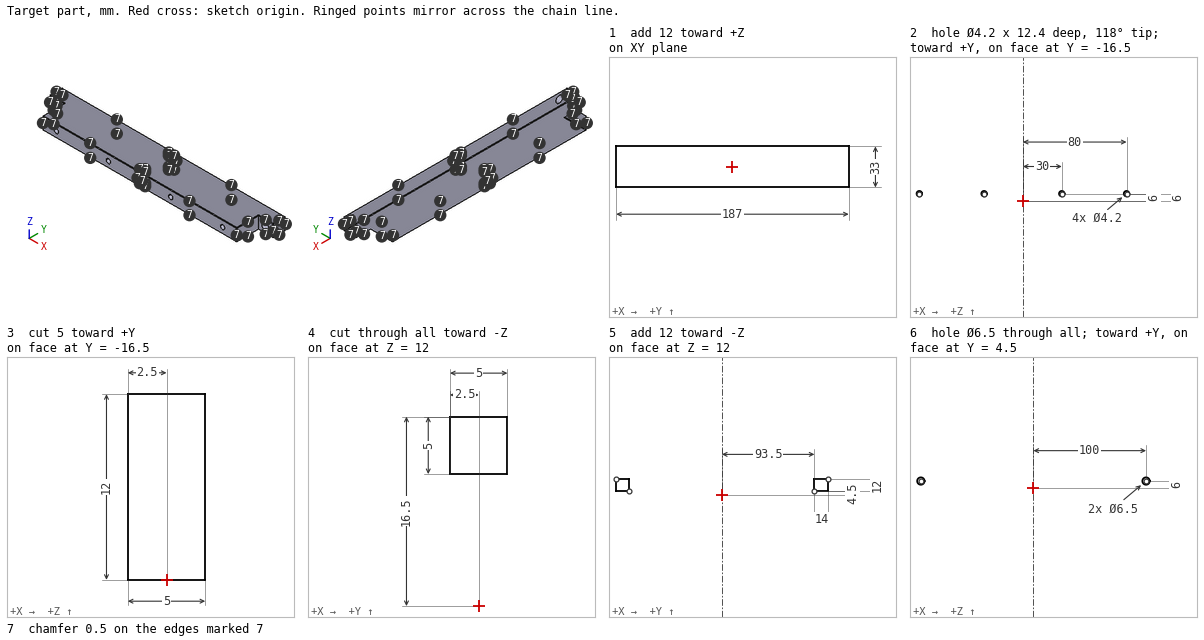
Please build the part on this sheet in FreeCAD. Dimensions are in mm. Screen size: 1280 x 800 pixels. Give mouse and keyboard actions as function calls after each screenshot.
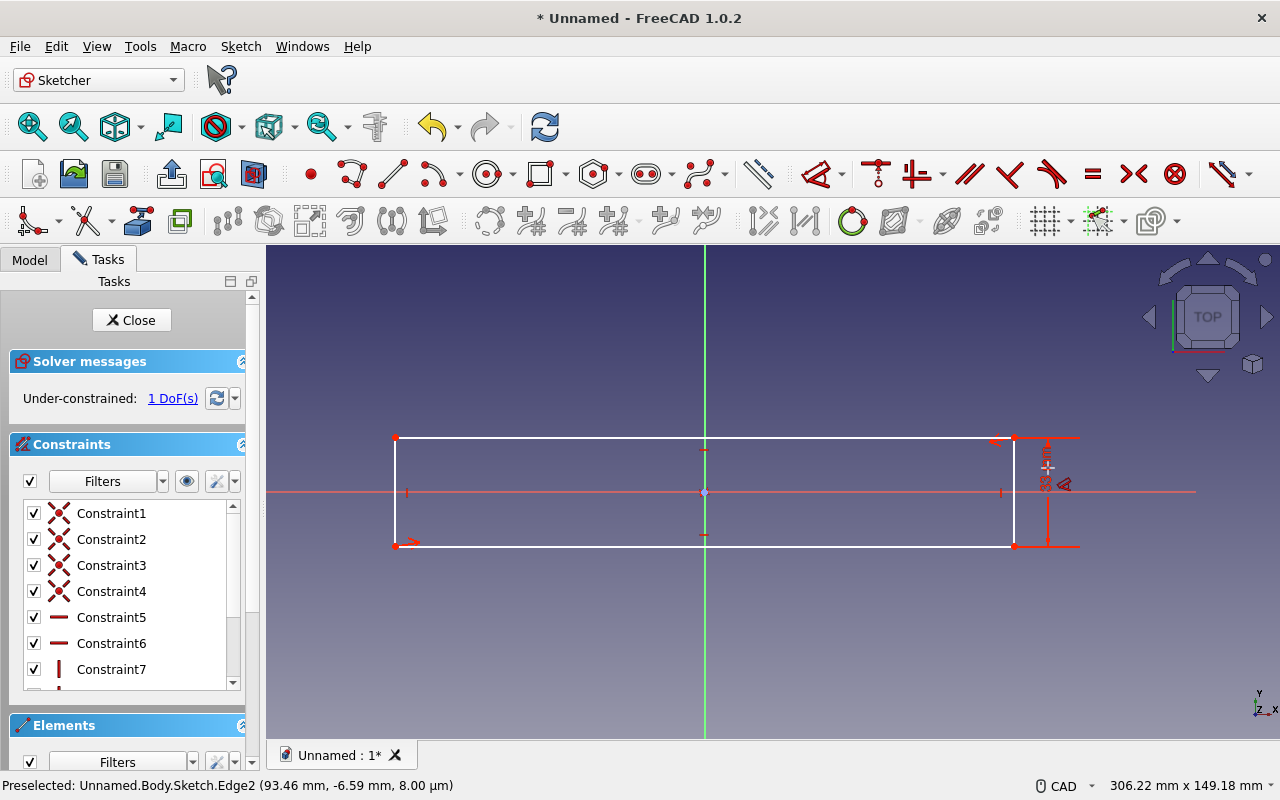
click(581, 547)
click(562, 581)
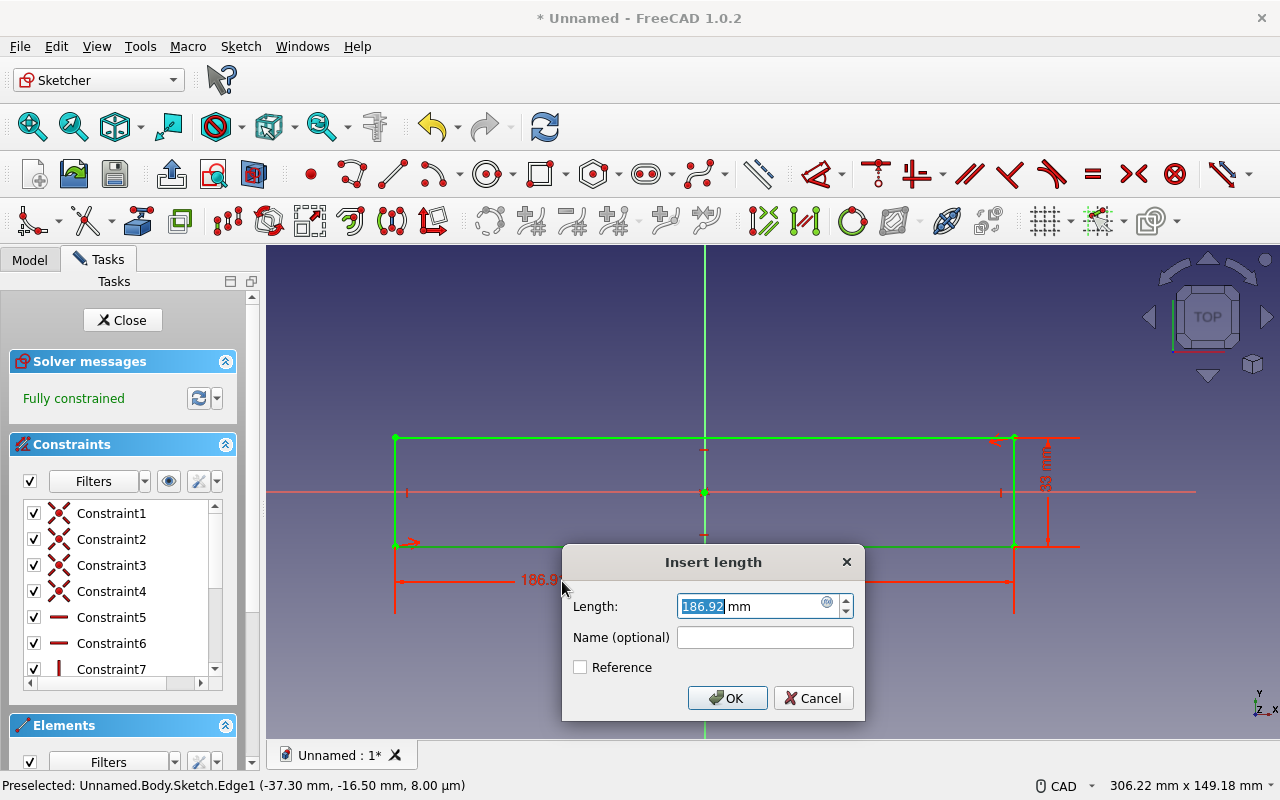
text(187)
key(Return)
key(Escape)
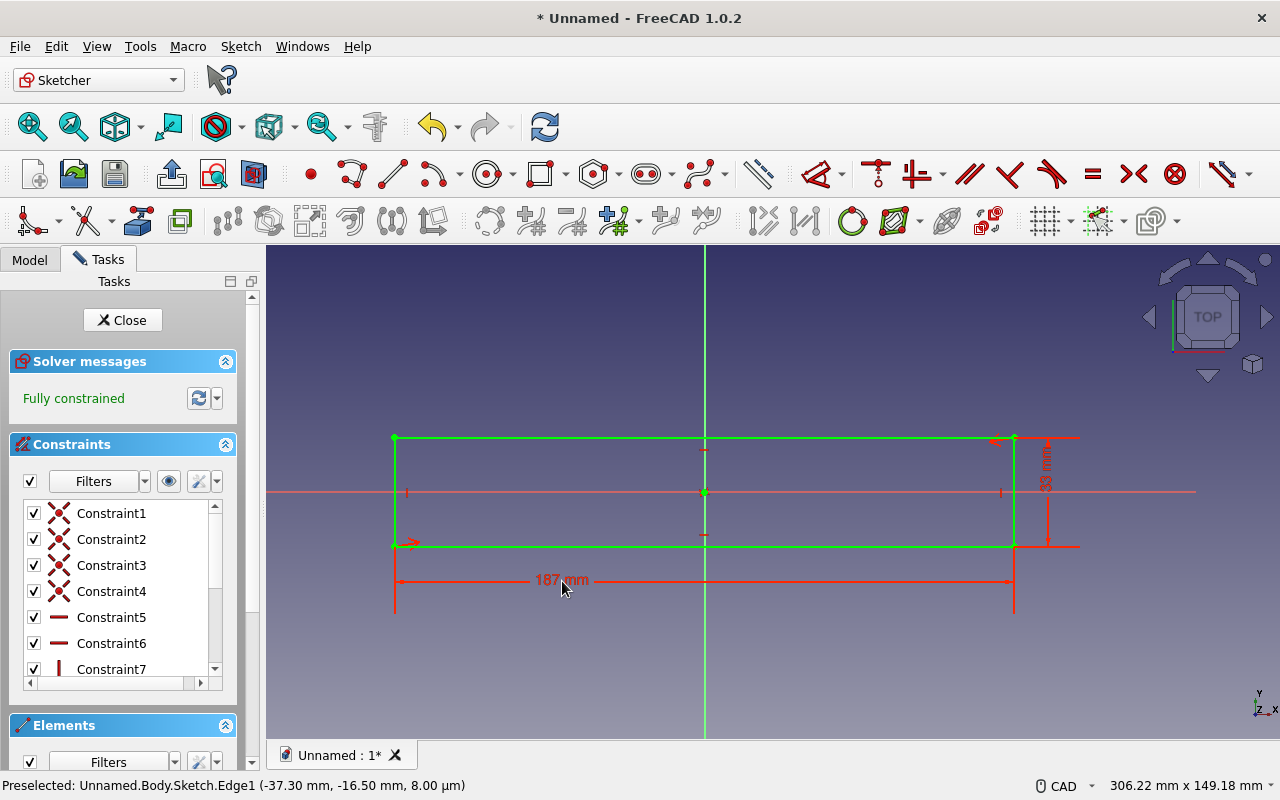
click(123, 320)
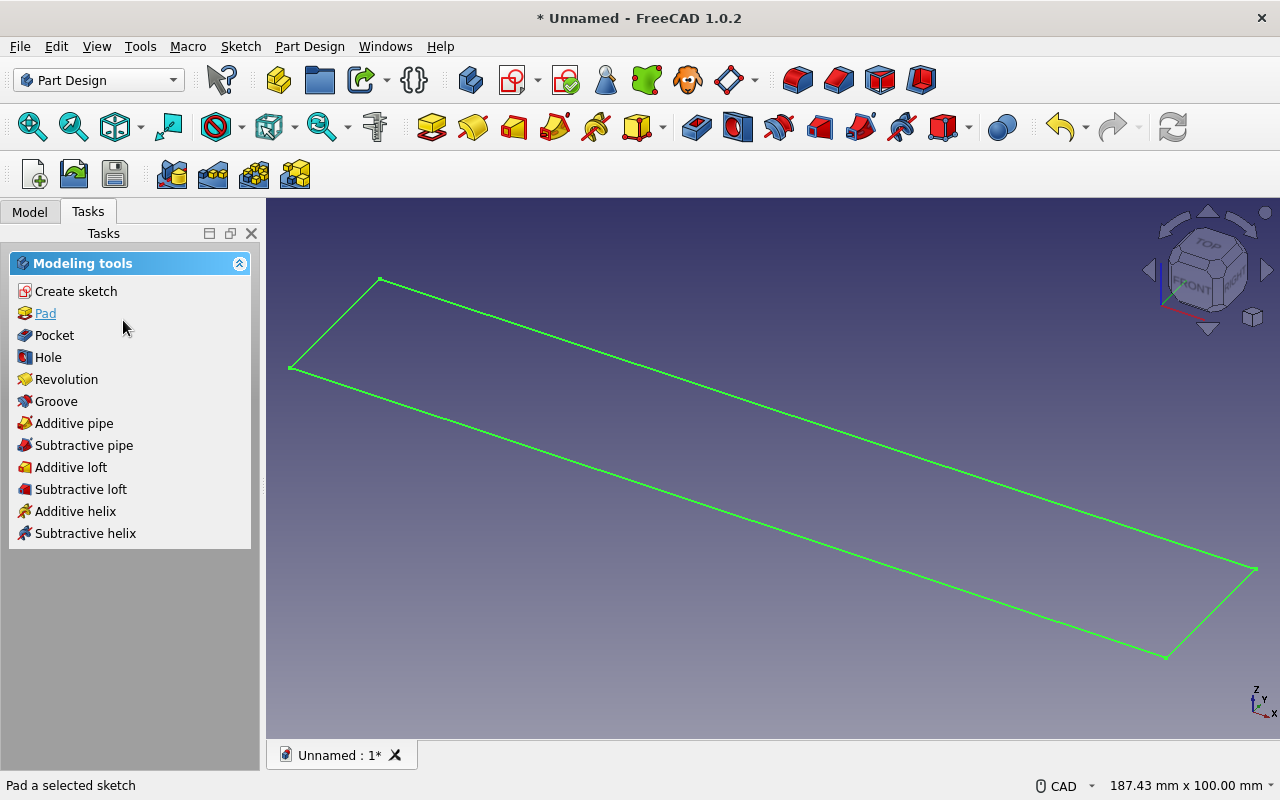
click(432, 128)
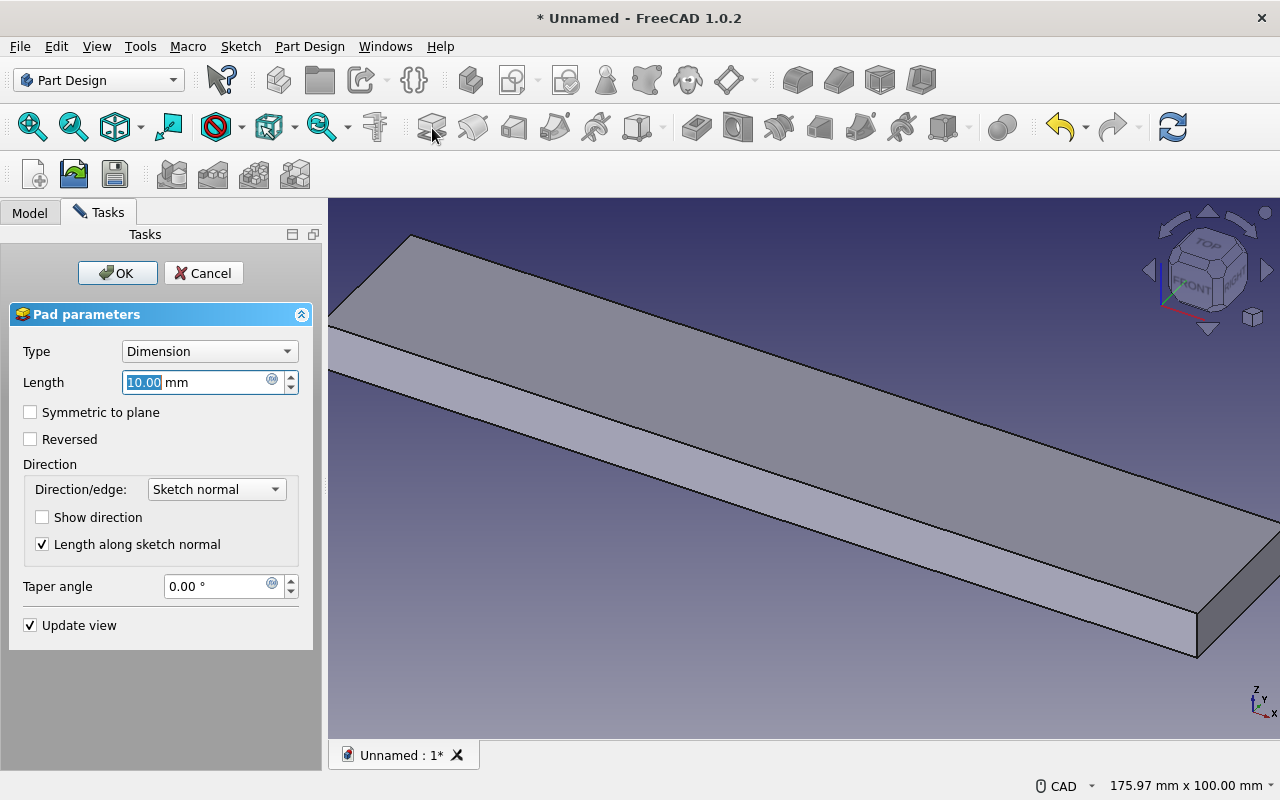
text(12)
key(Tab)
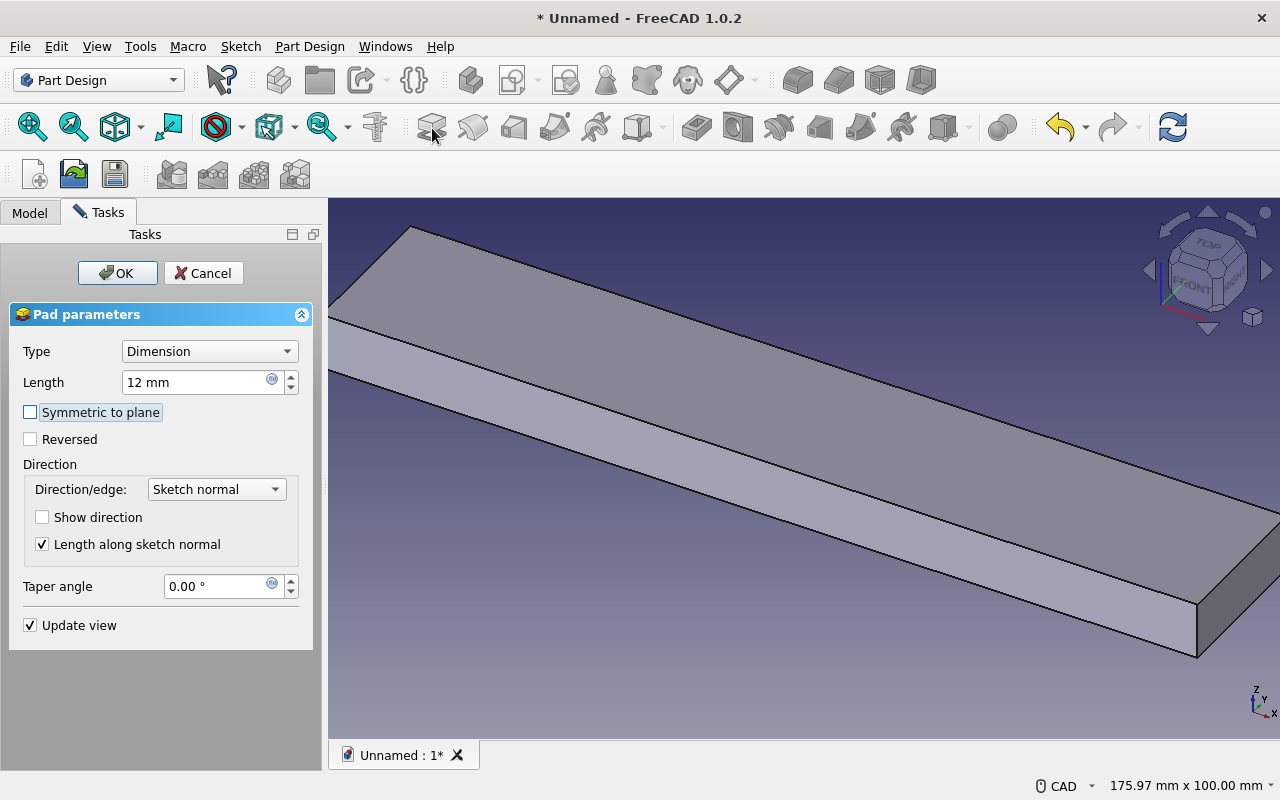
click(118, 273)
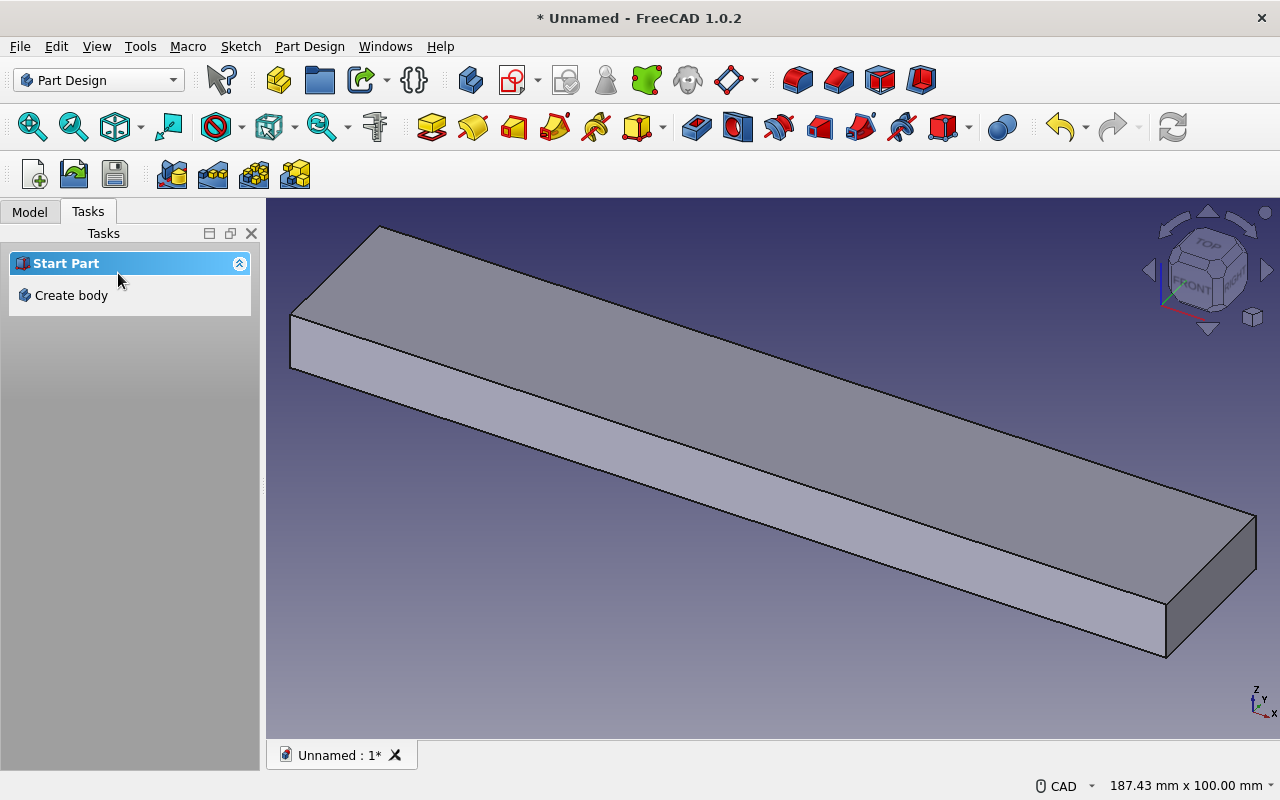
click(1104, 610)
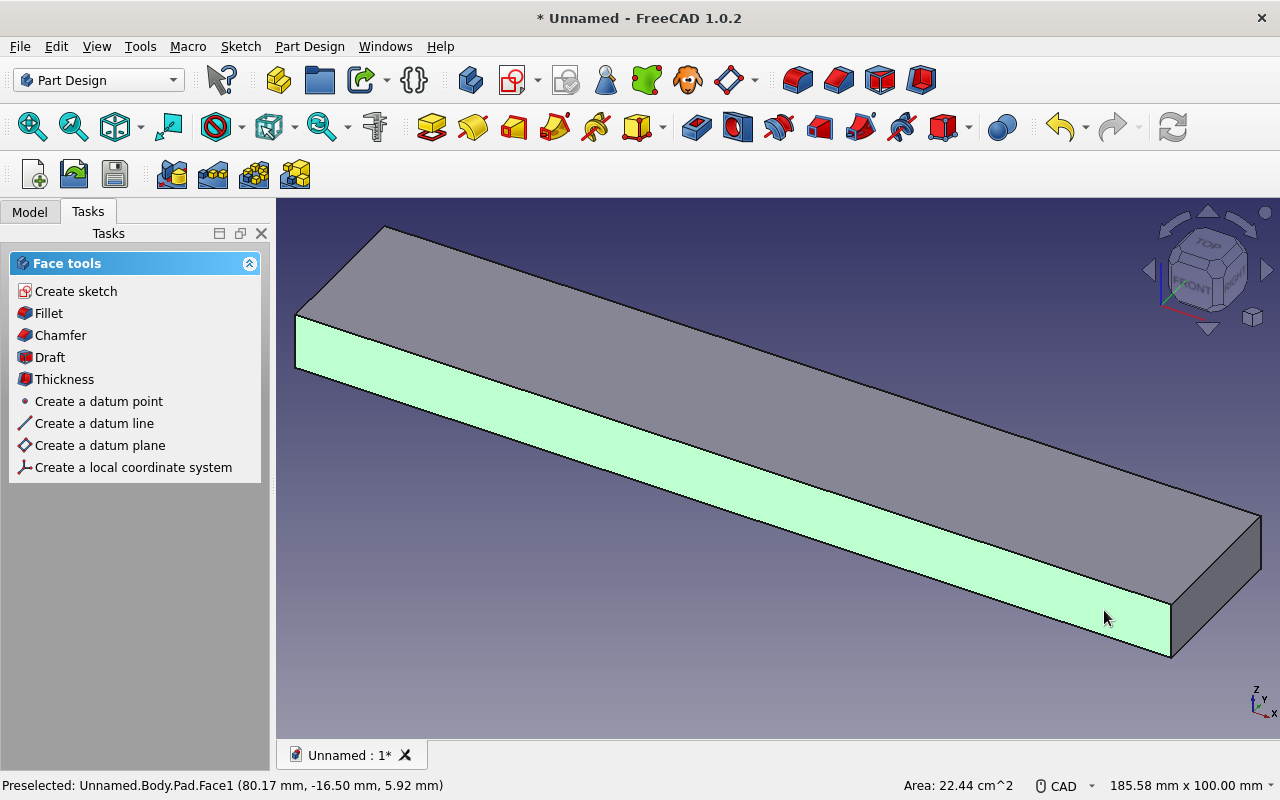
click(512, 80)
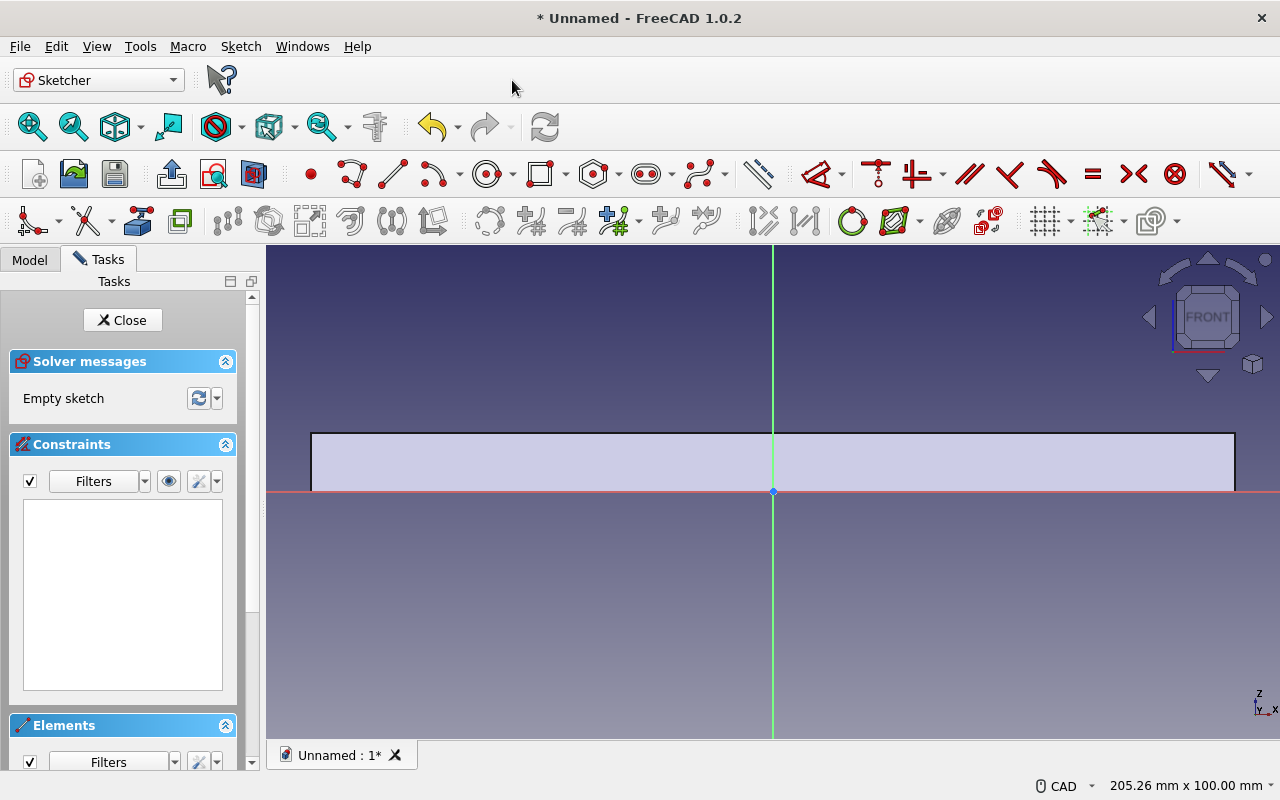
scroll(565, 533, down, 2)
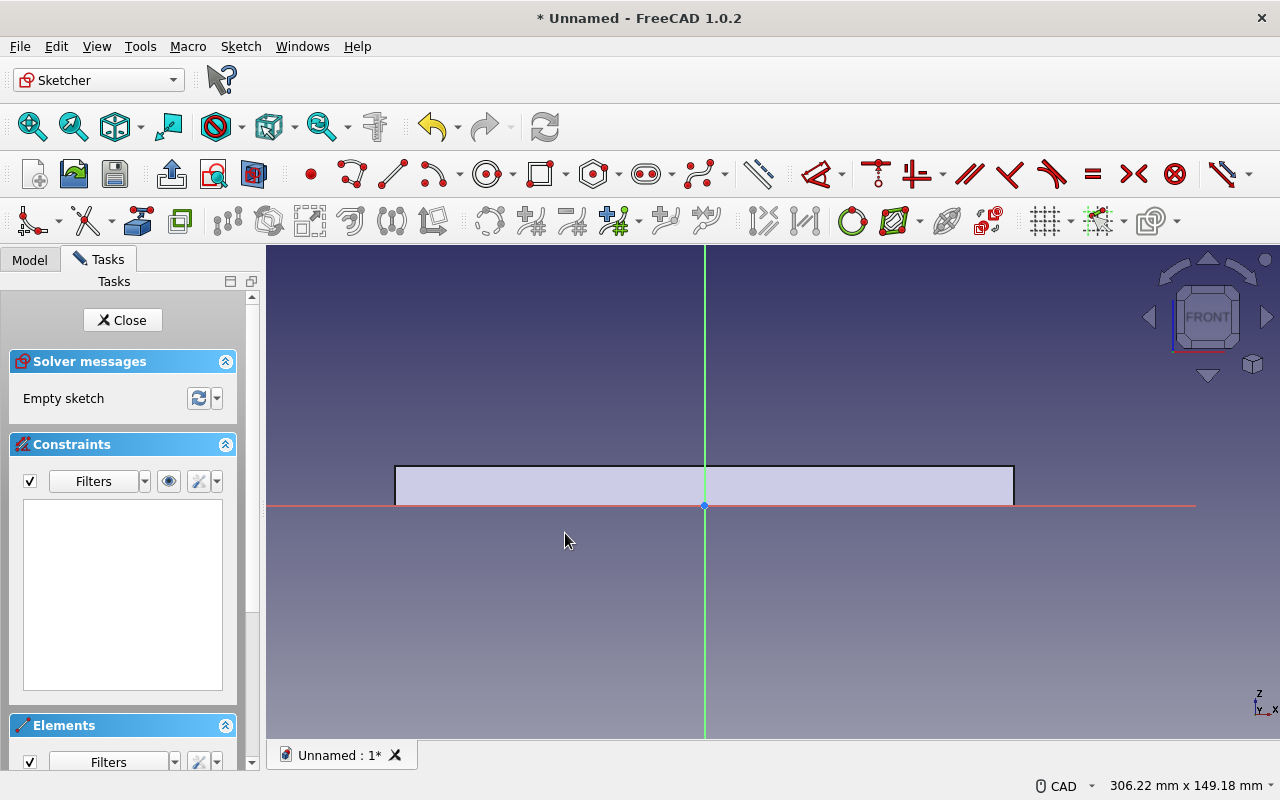
key(g)
key(c)